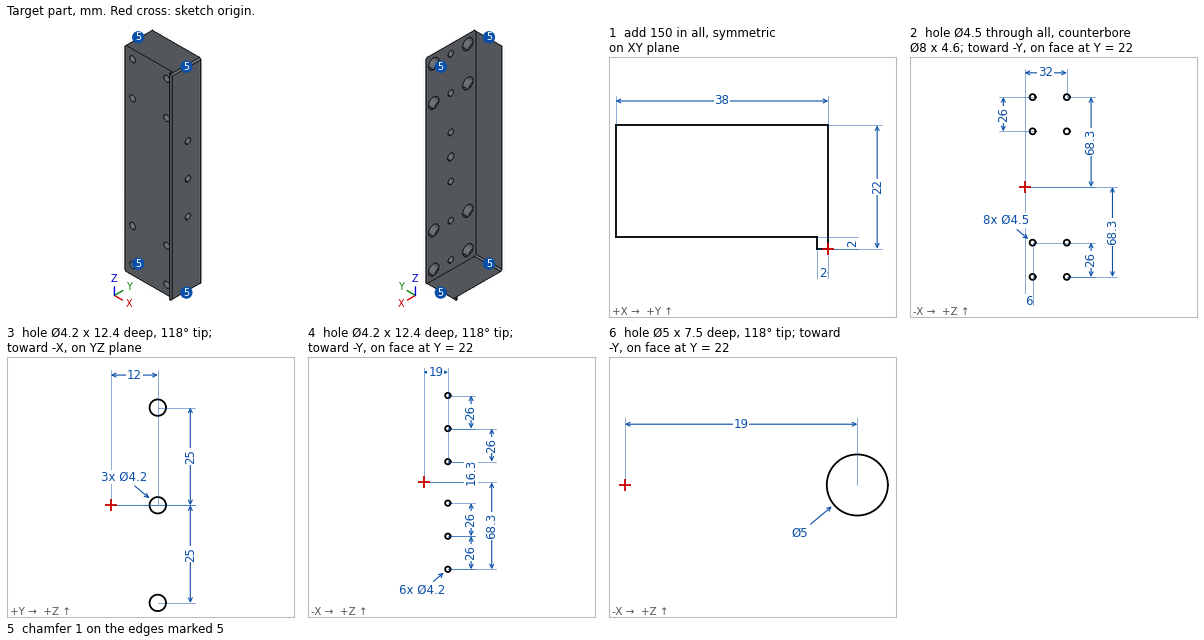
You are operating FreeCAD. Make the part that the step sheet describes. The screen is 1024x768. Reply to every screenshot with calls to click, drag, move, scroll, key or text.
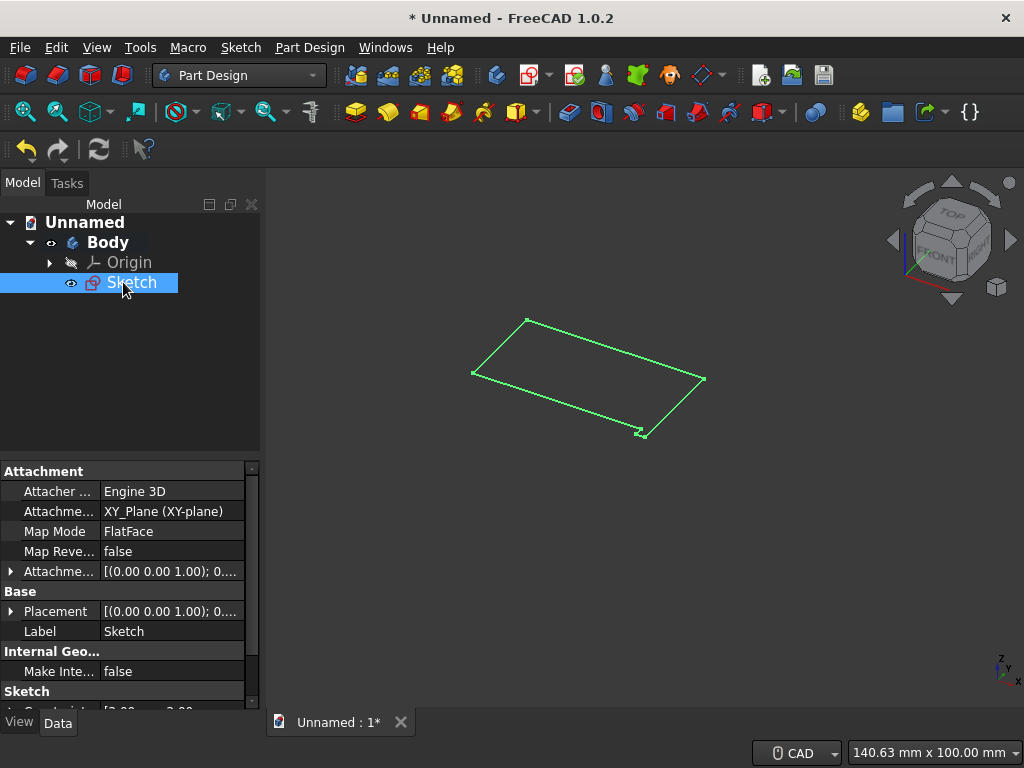
click(356, 112)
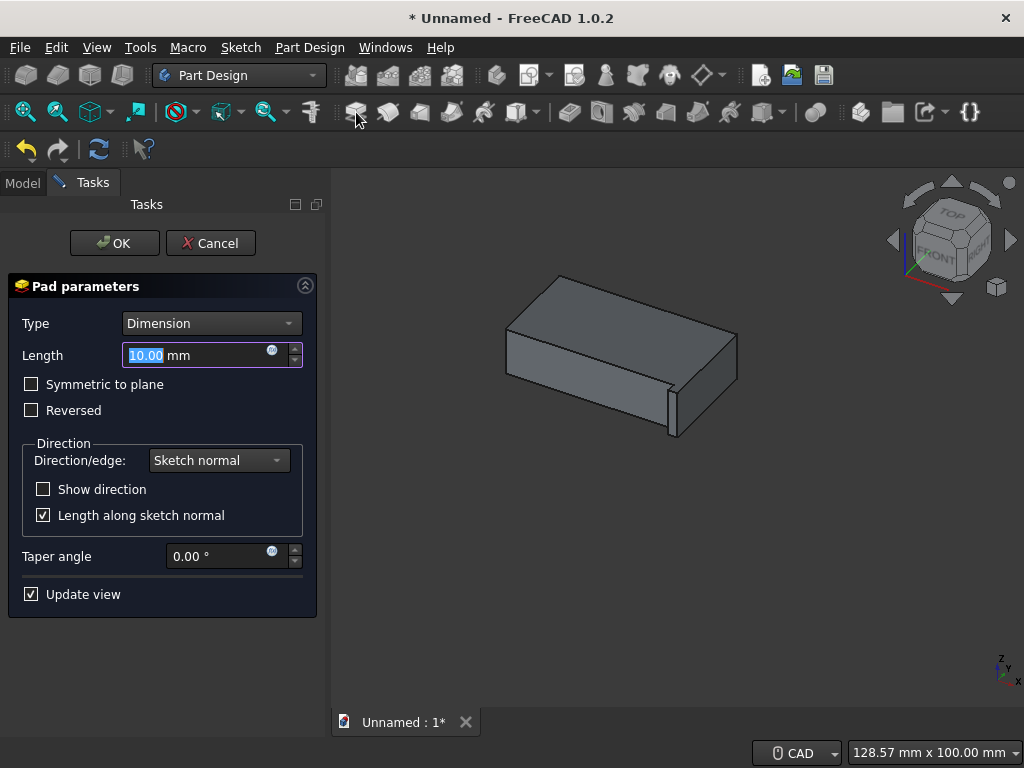
text(150)
key(Tab)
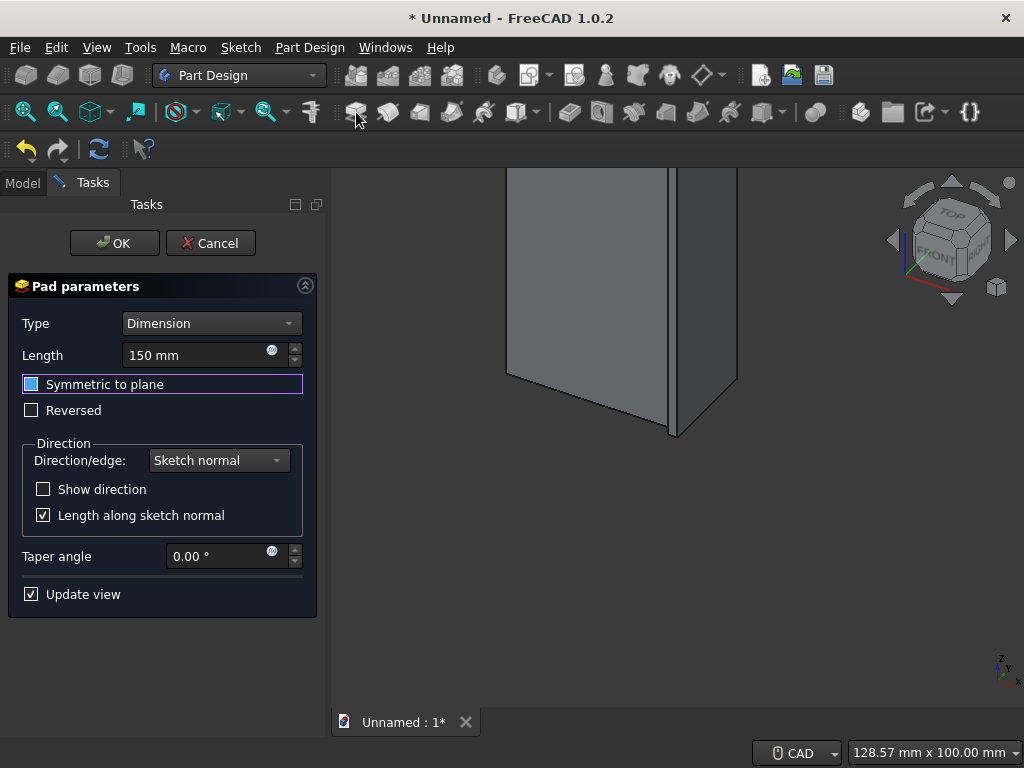
click(30, 384)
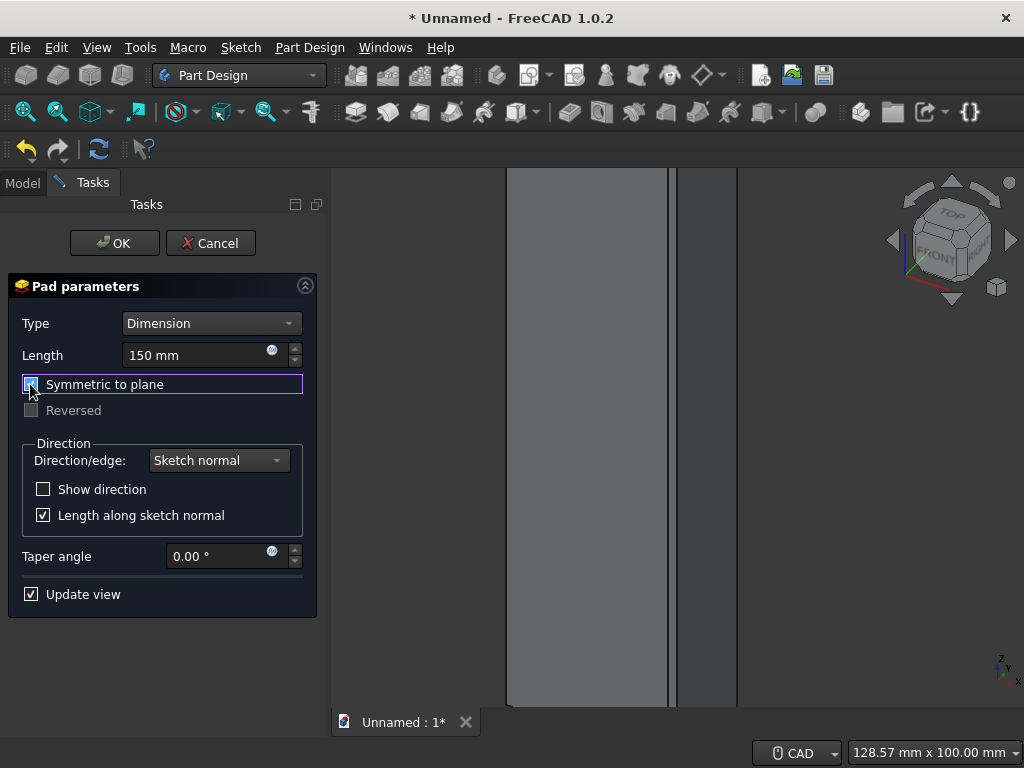
click(115, 243)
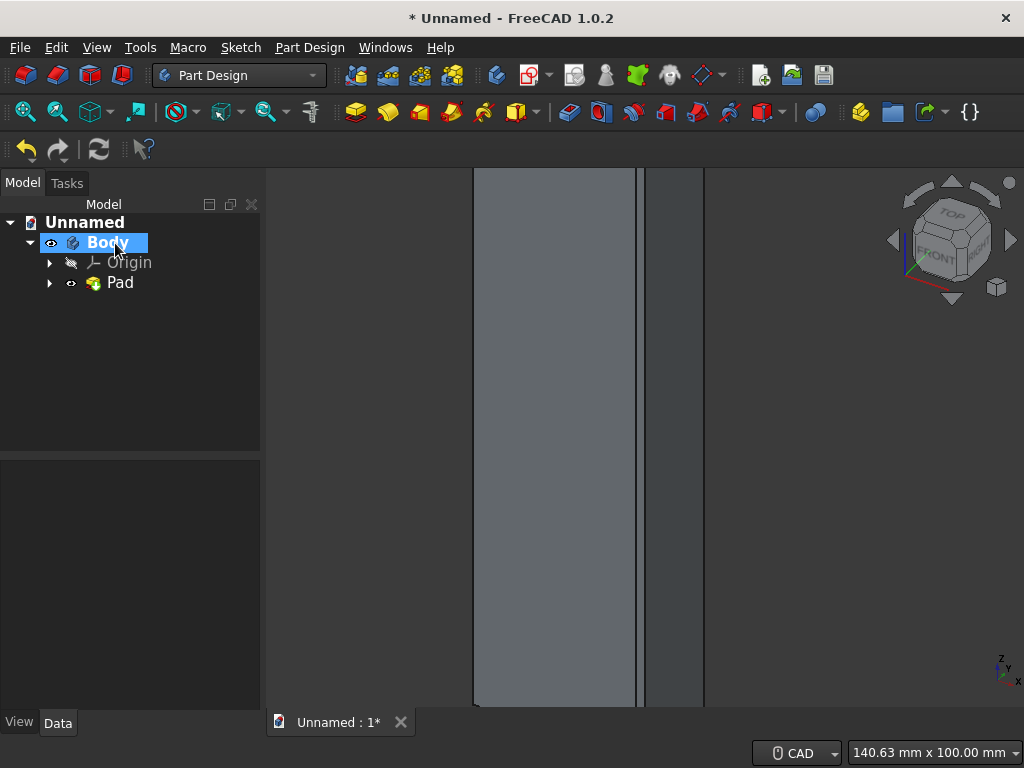
key(v)
key(f)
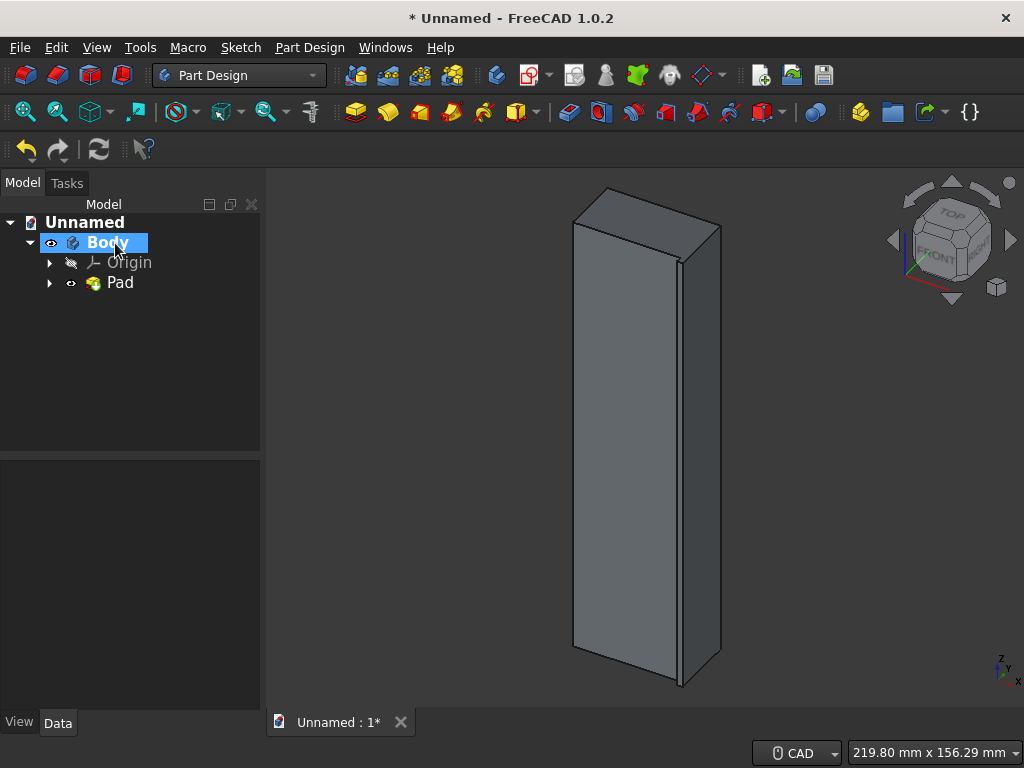
key(4)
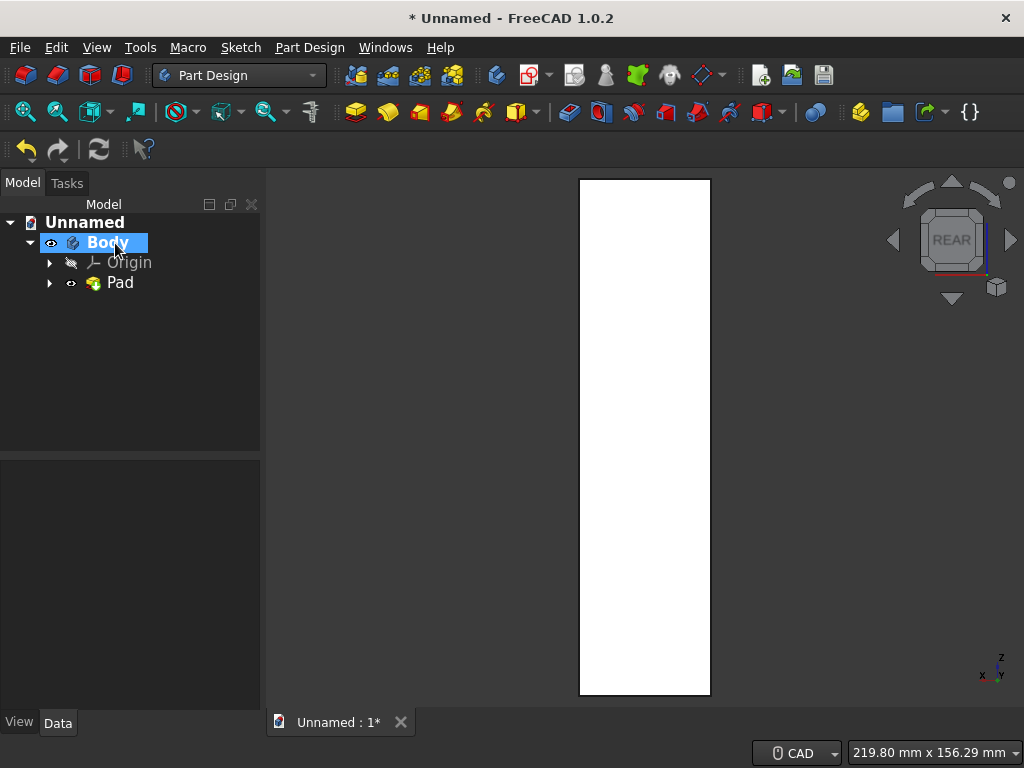
click(645, 289)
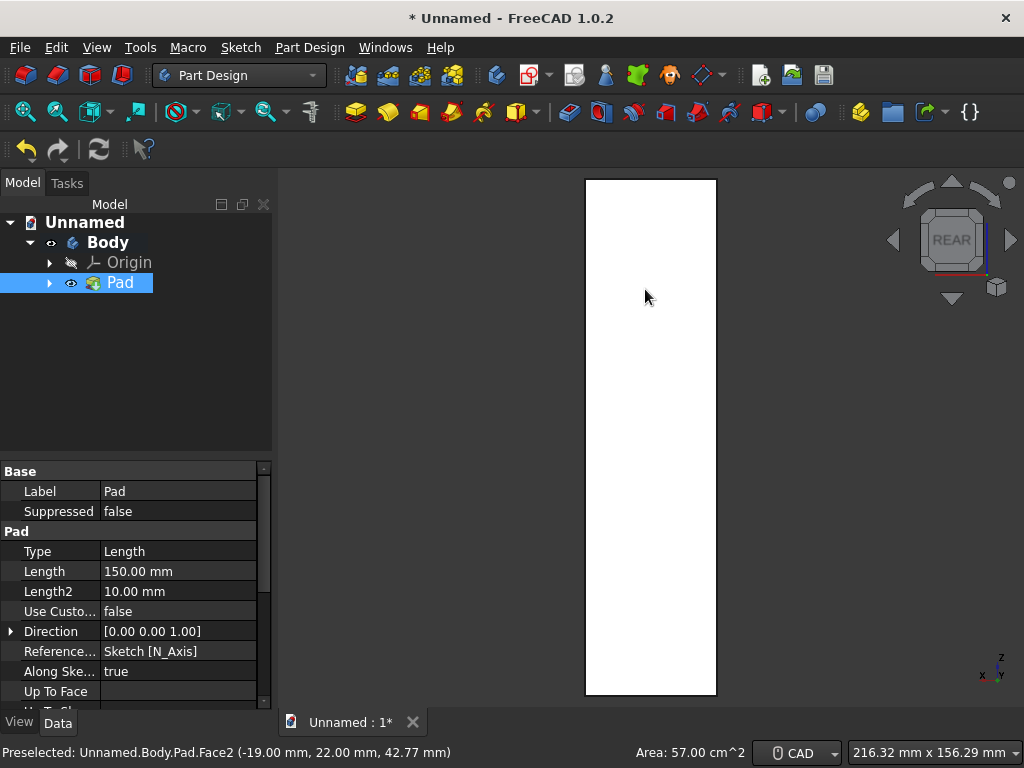
click(530, 76)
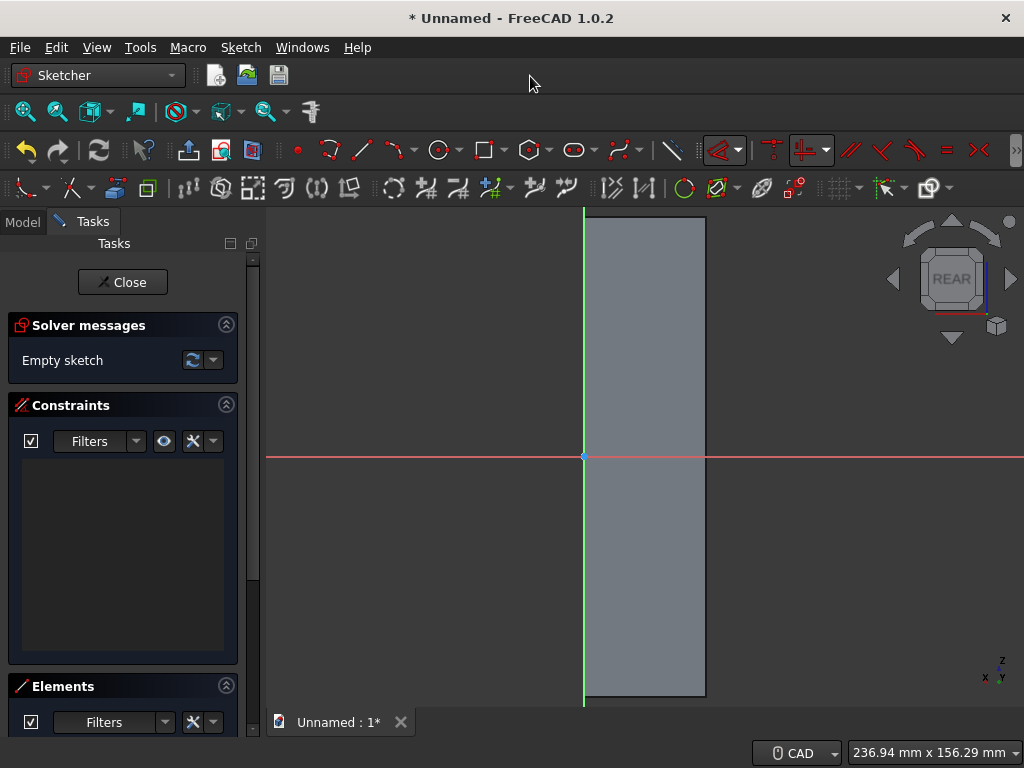
scroll(449, 457, down, 2)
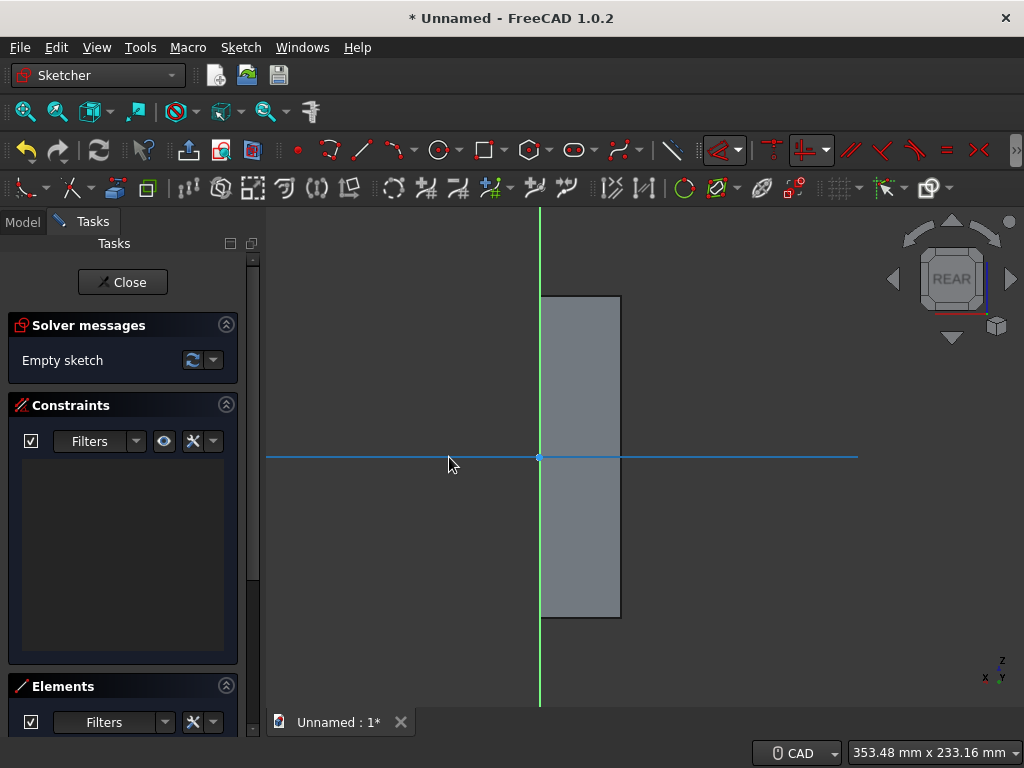
key(g)
key(c)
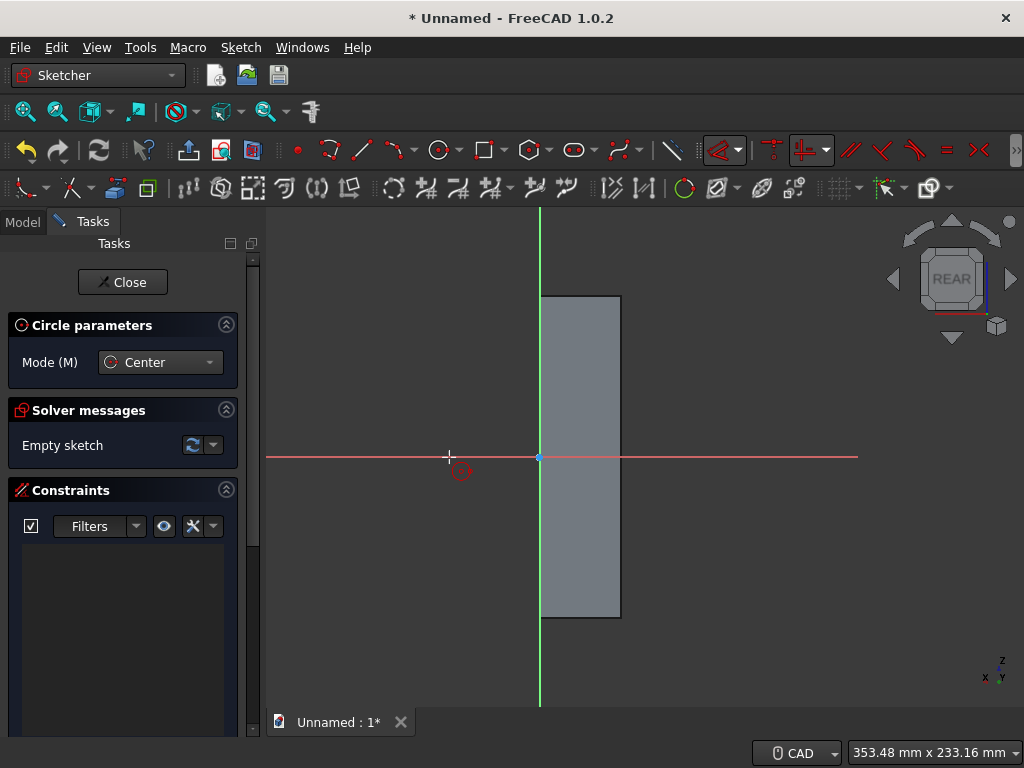
scroll(608, 311, up, 8)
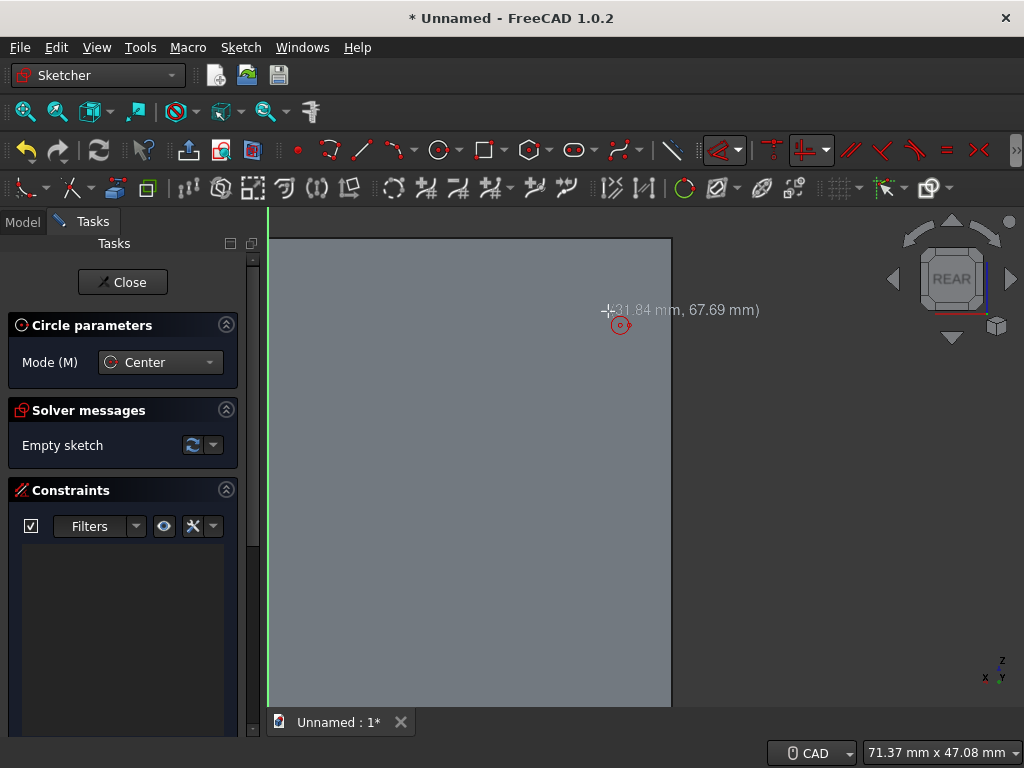
scroll(609, 311, down, 8)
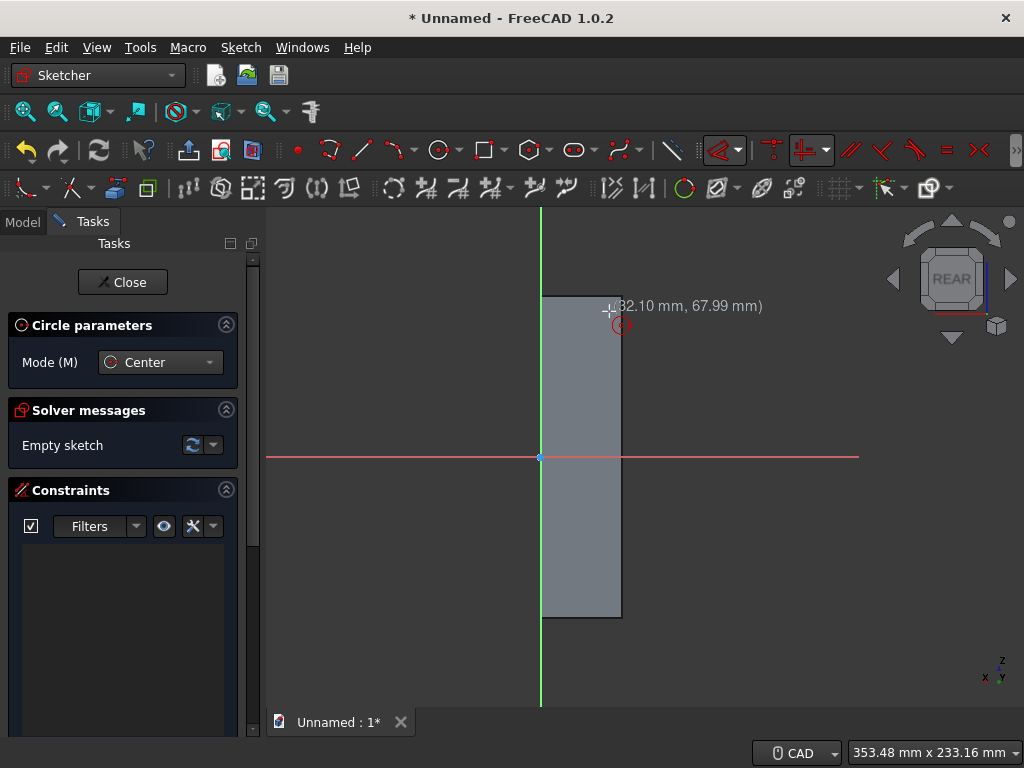
click(609, 311)